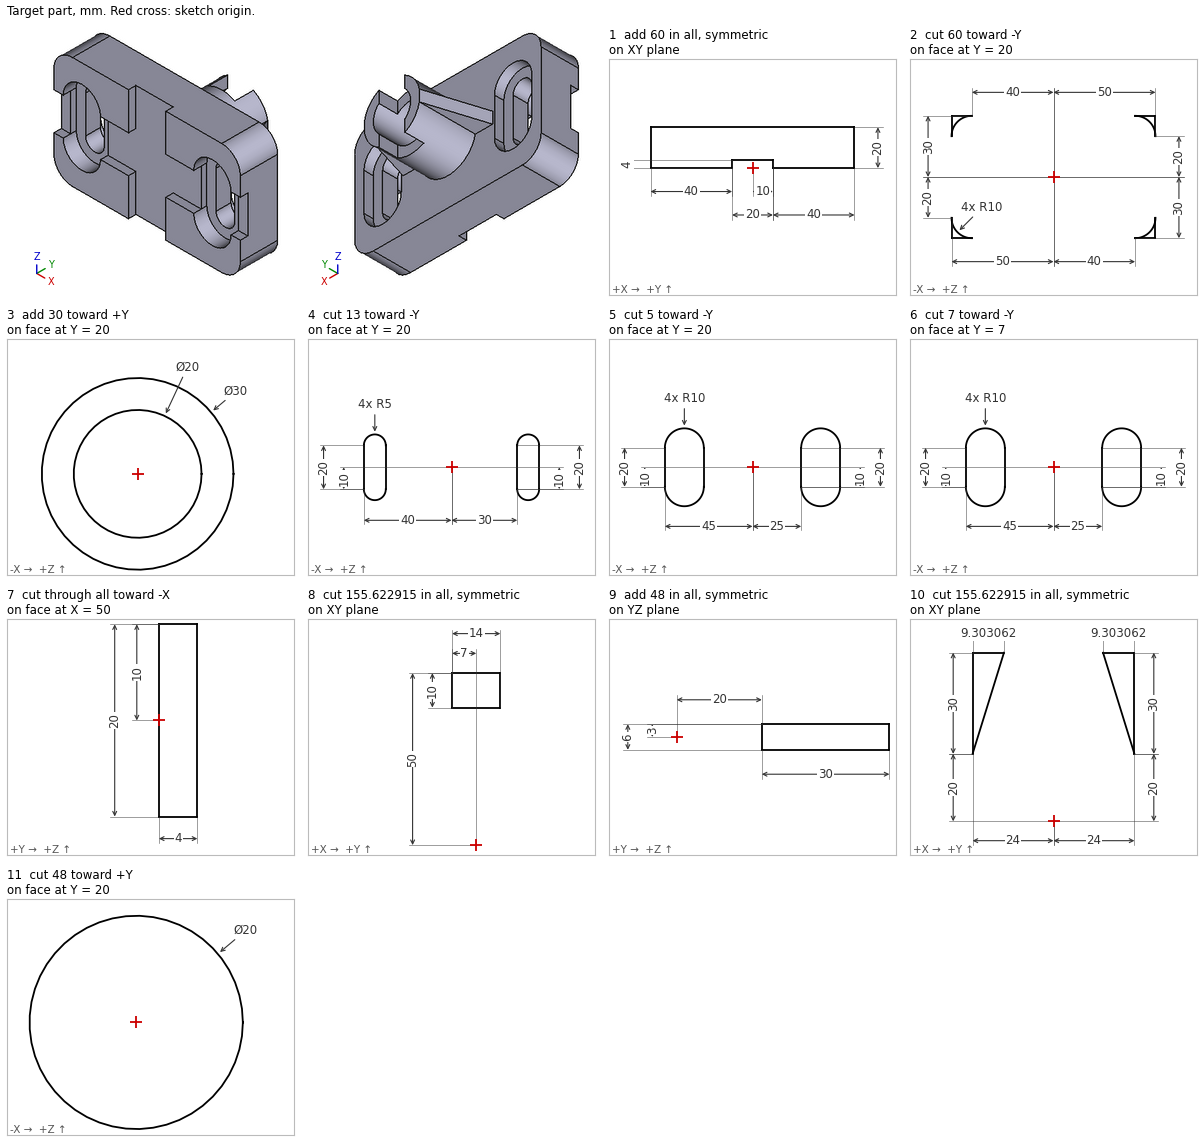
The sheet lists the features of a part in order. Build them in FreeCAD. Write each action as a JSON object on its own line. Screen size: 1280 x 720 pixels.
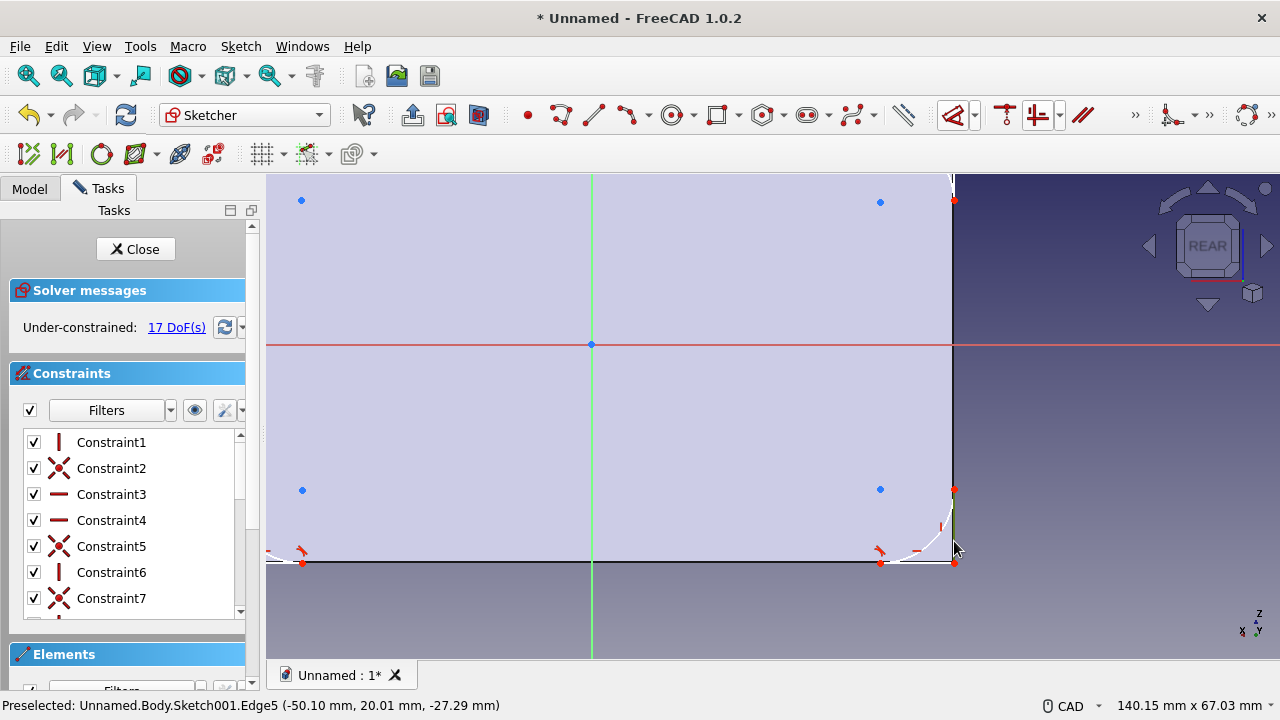
{"action": "left_click", "coordinate": [932, 542]}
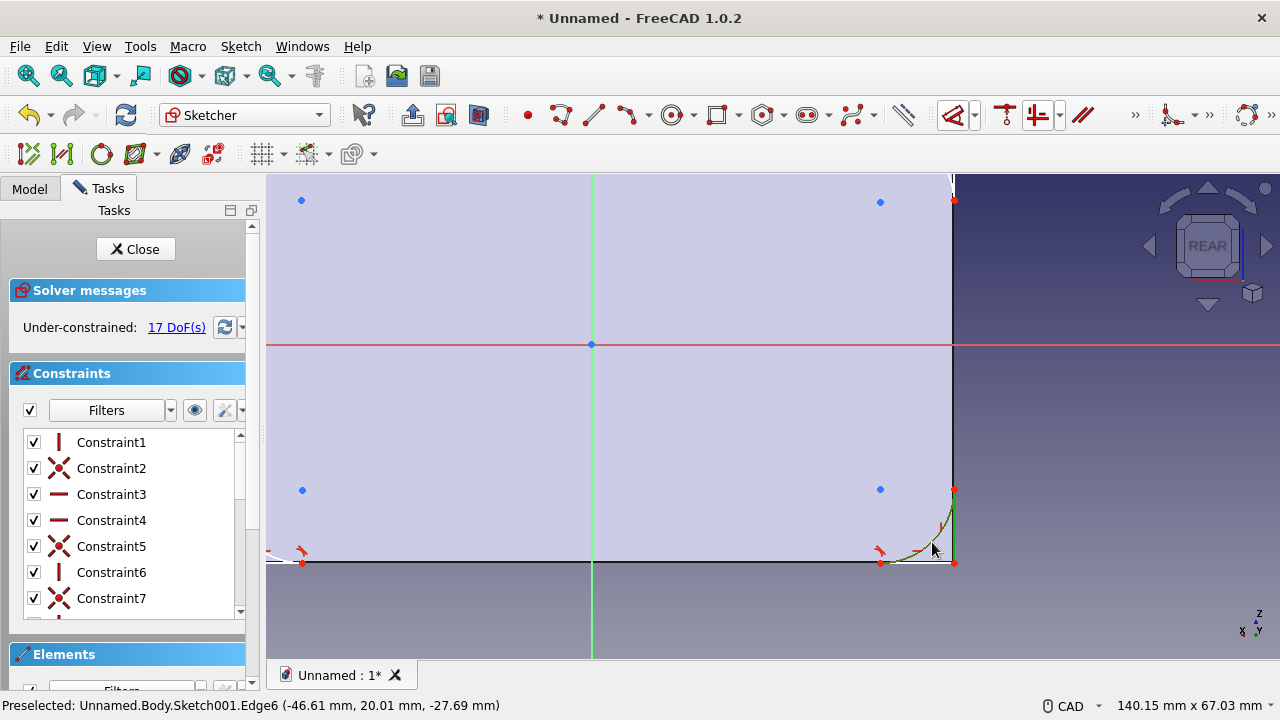
{"action": "key", "text": "t"}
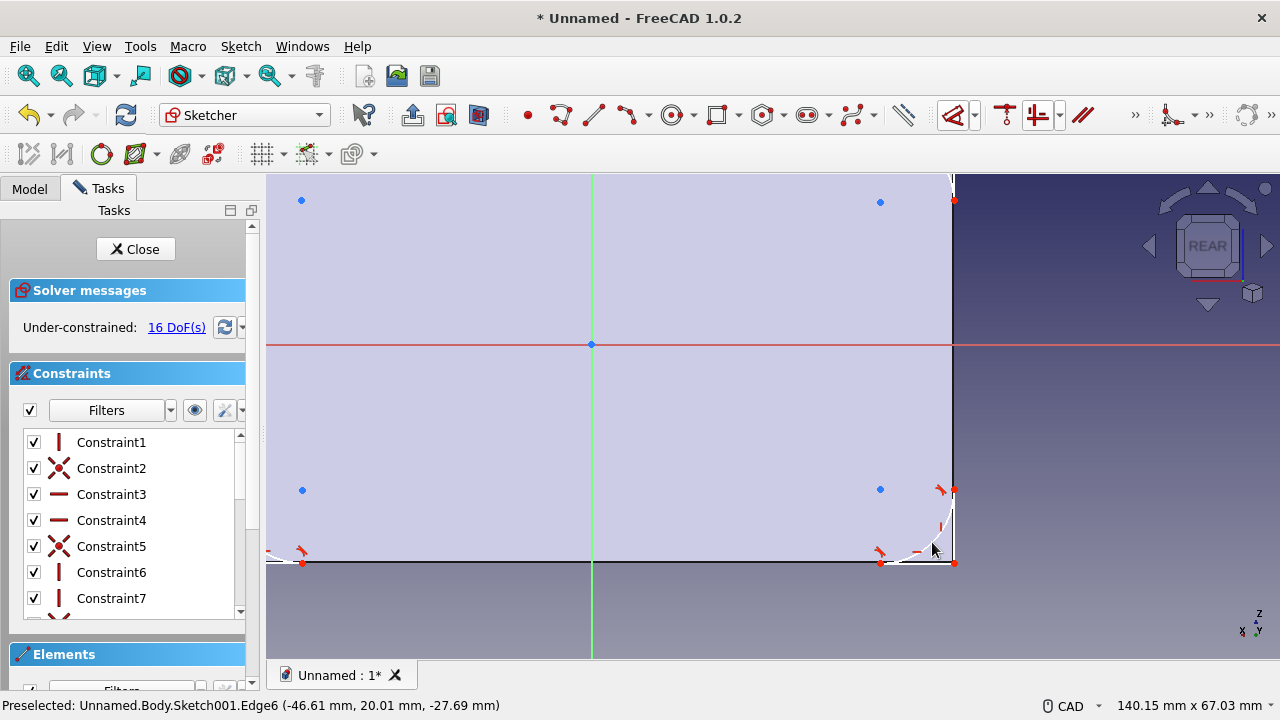
{"action": "scroll", "coordinate": [934, 563], "scroll_direction": "down", "scroll_amount": 2}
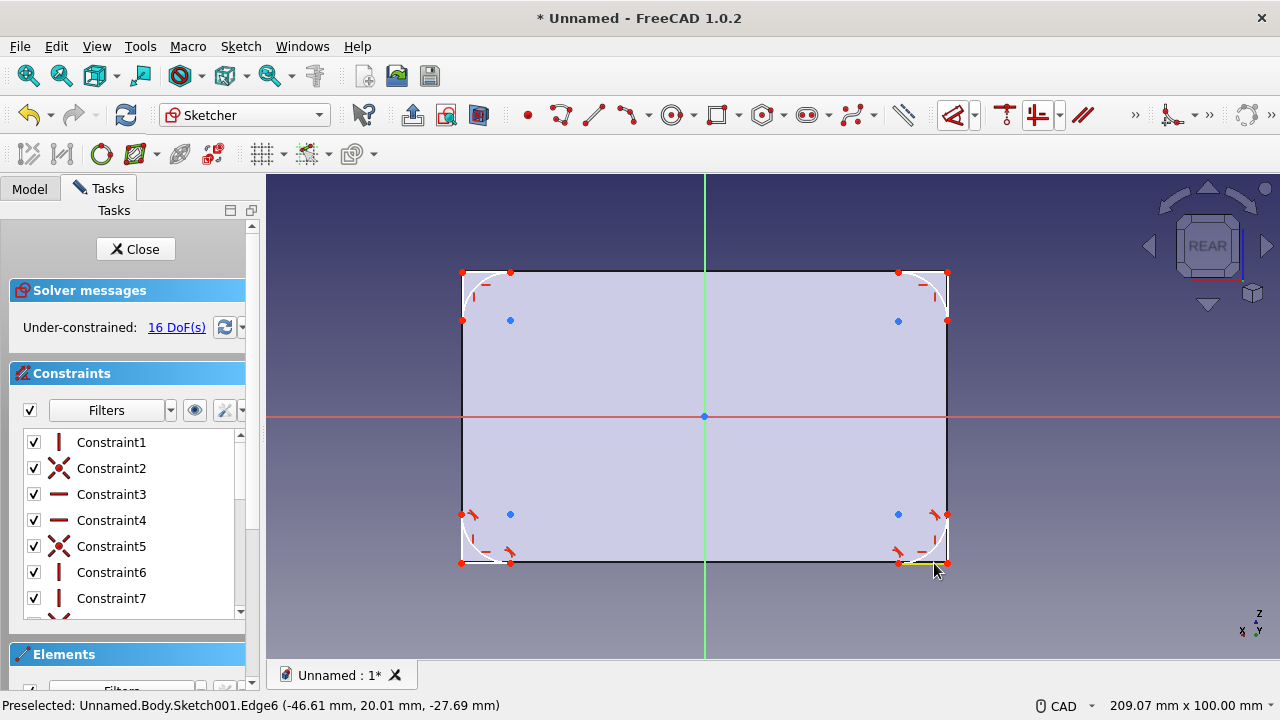
{"action": "scroll", "coordinate": [948, 287], "scroll_direction": "up", "scroll_amount": 2}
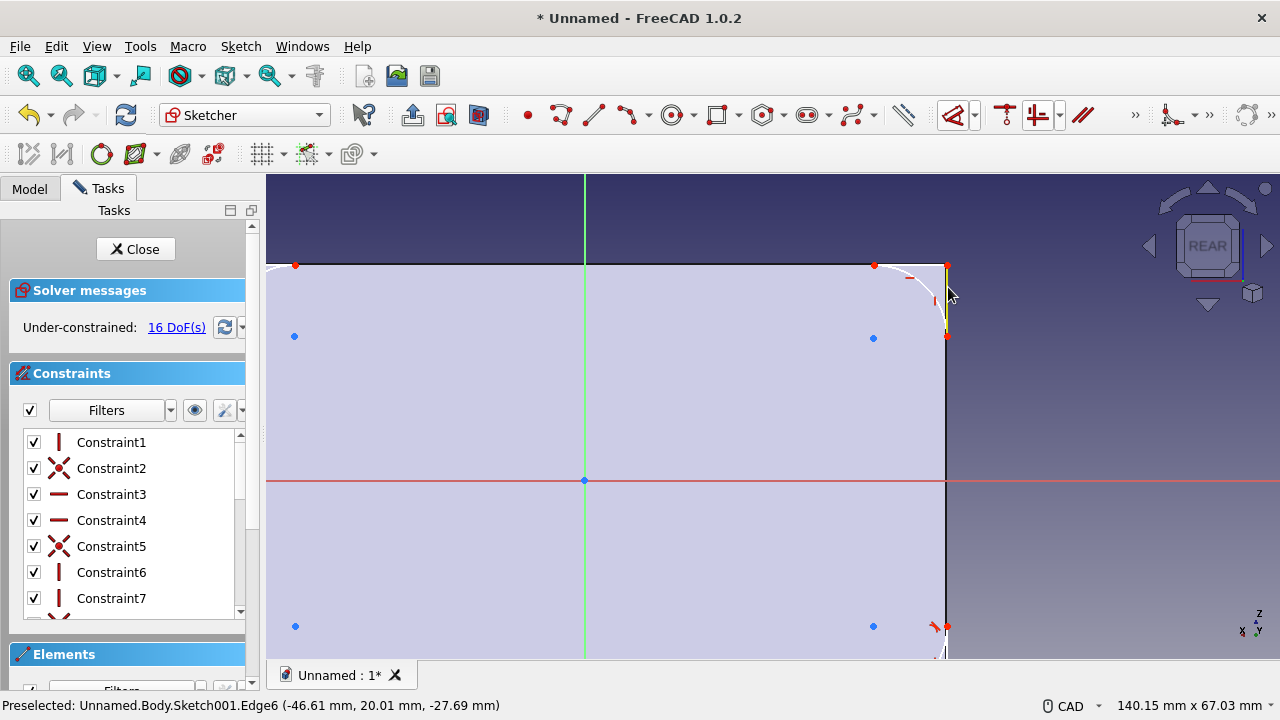
{"action": "left_click", "coordinate": [947, 286]}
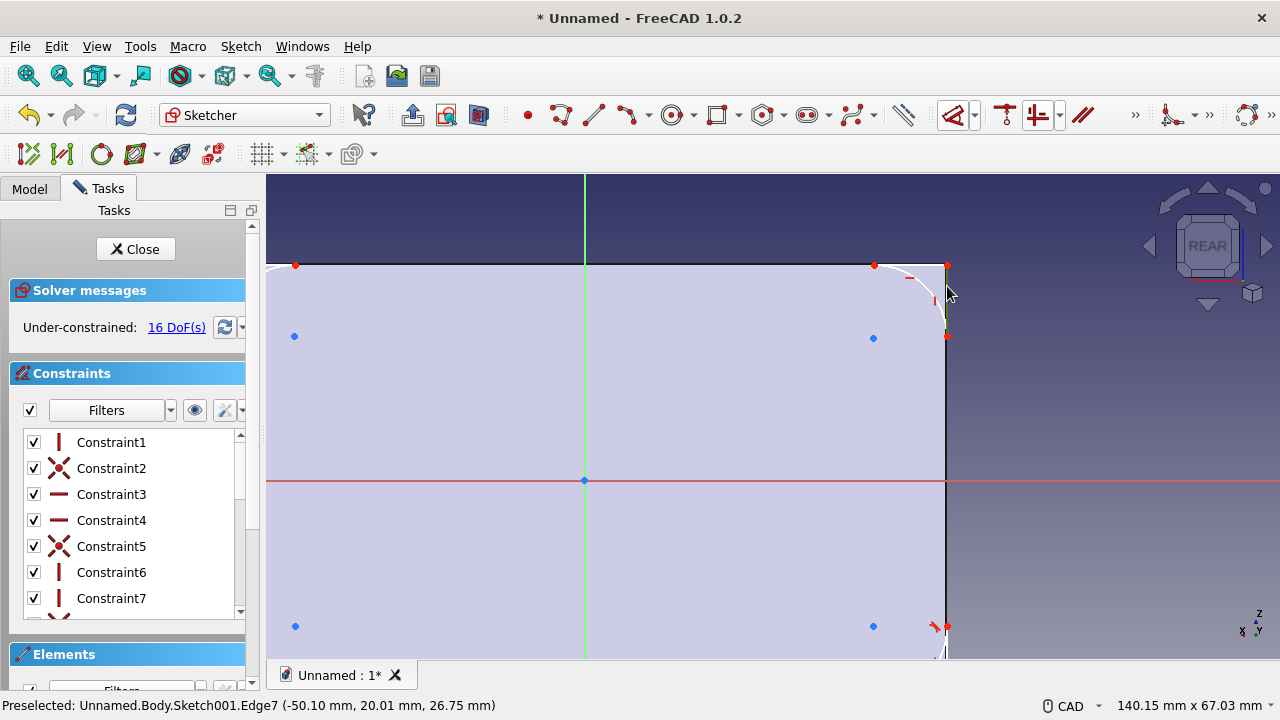
{"action": "left_click", "coordinate": [925, 286]}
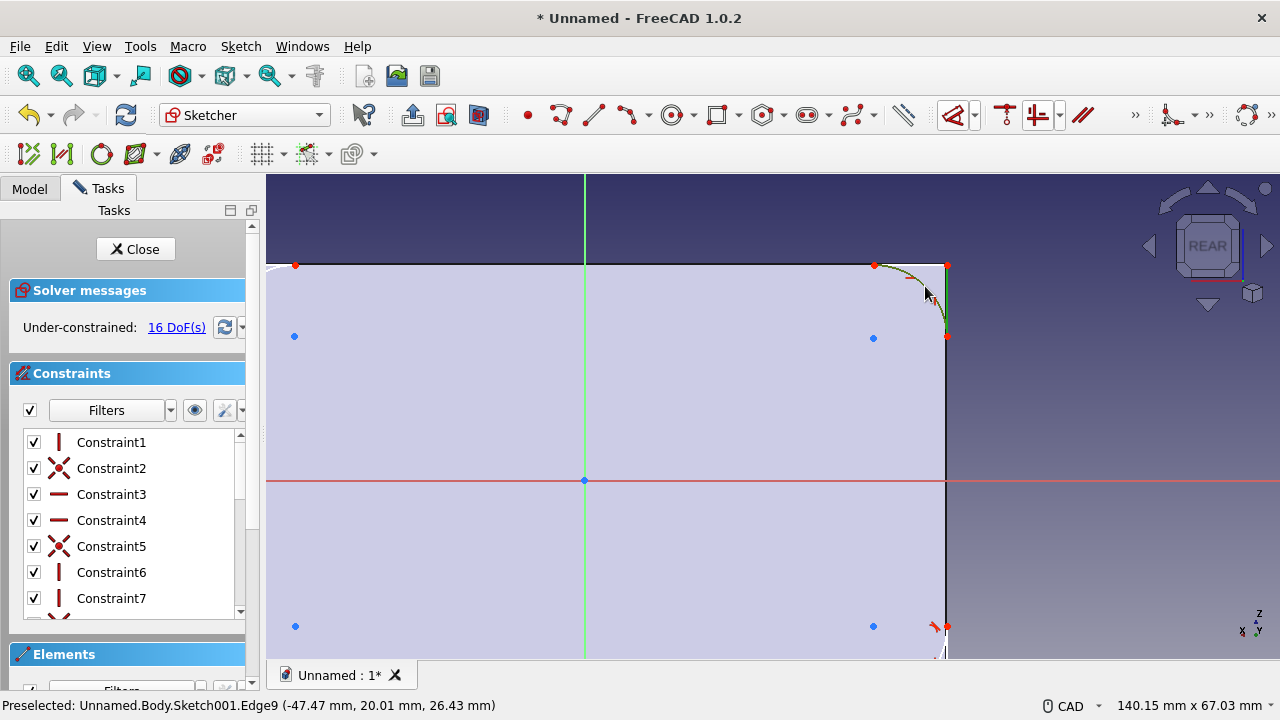
{"action": "key", "text": "t"}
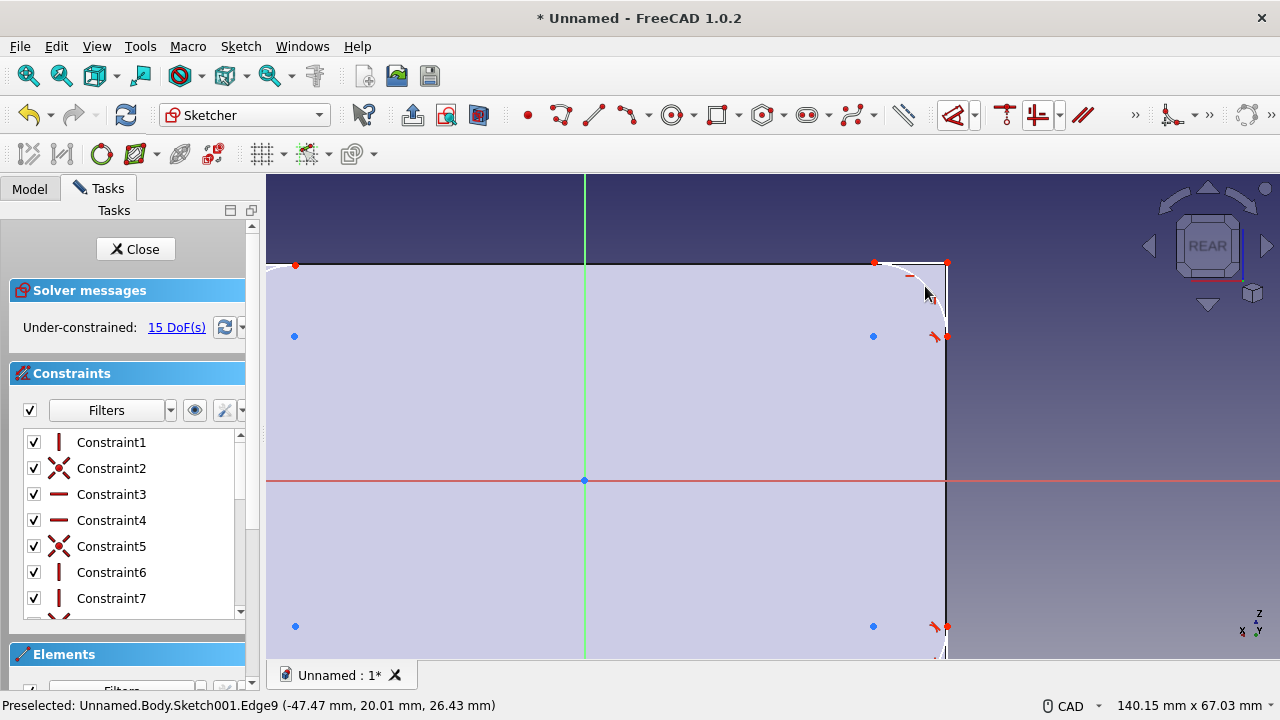
{"action": "left_click", "coordinate": [925, 263]}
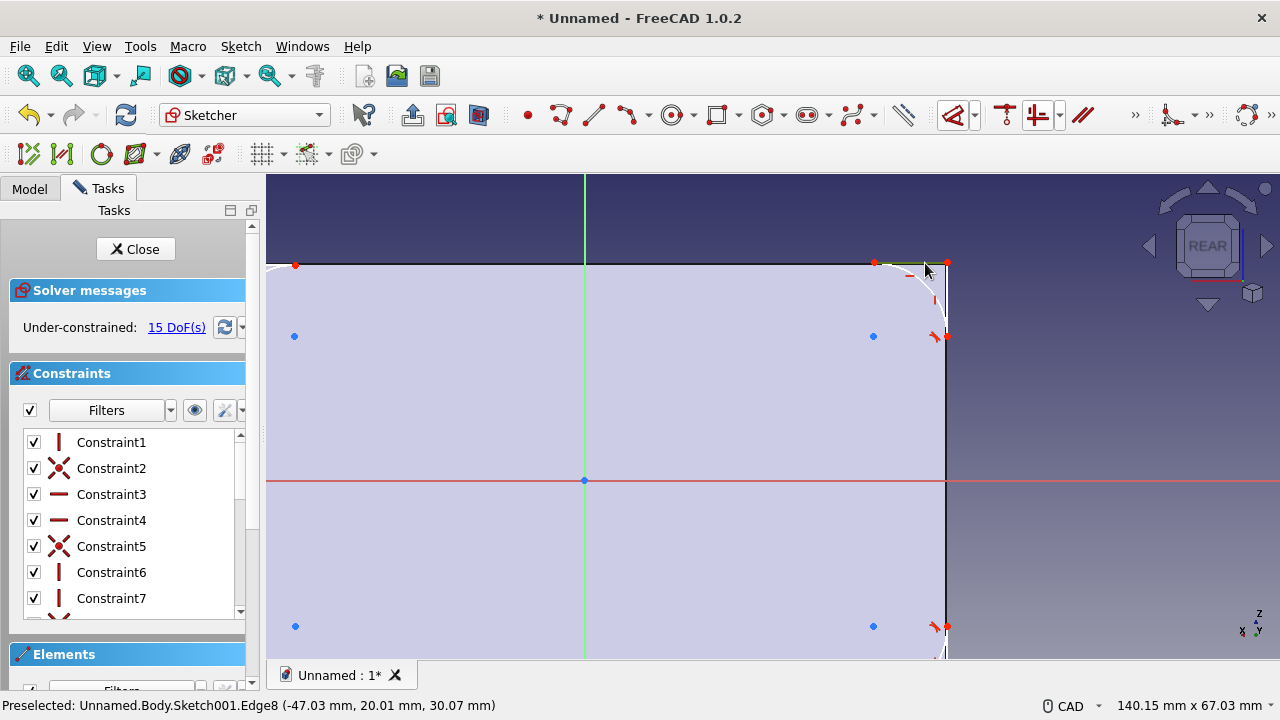
{"action": "left_click", "coordinate": [926, 285]}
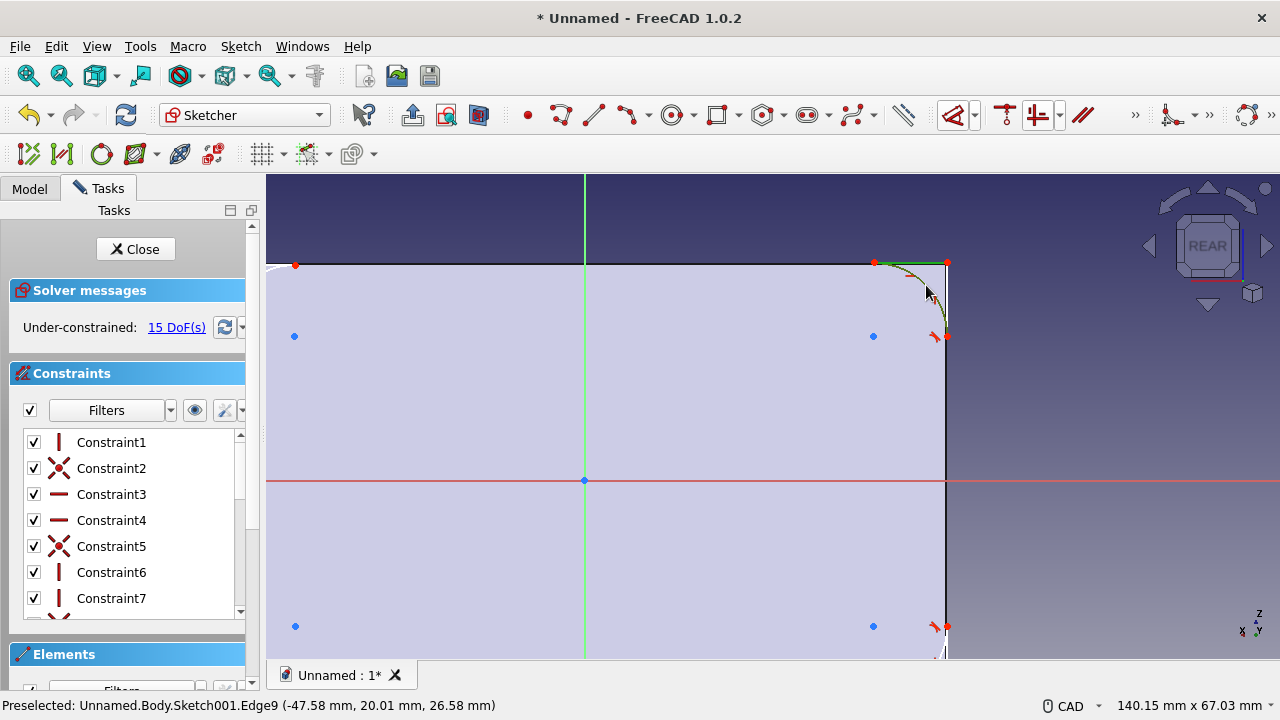
{"action": "key", "text": "t"}